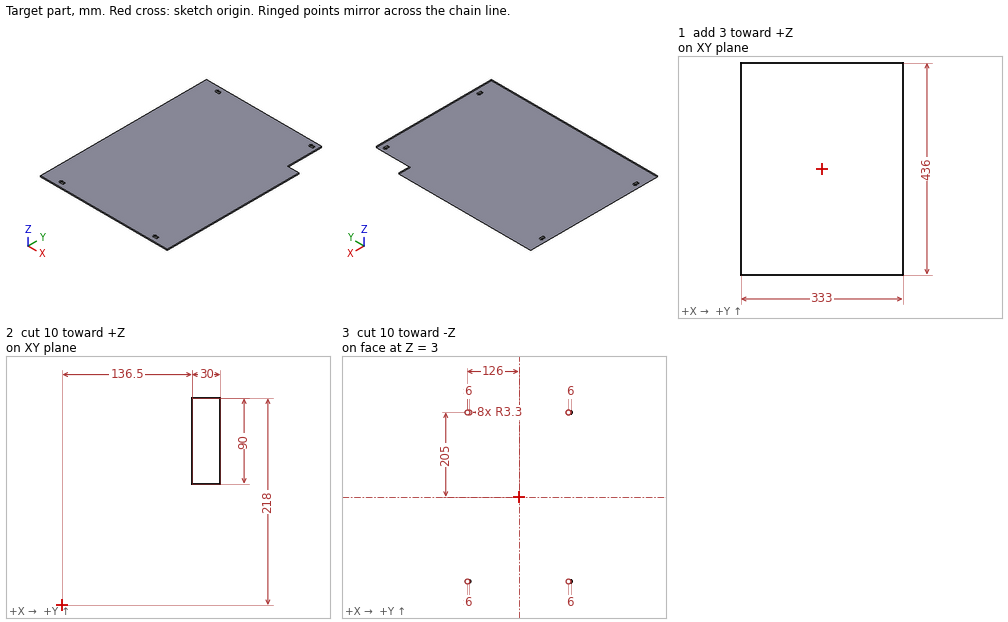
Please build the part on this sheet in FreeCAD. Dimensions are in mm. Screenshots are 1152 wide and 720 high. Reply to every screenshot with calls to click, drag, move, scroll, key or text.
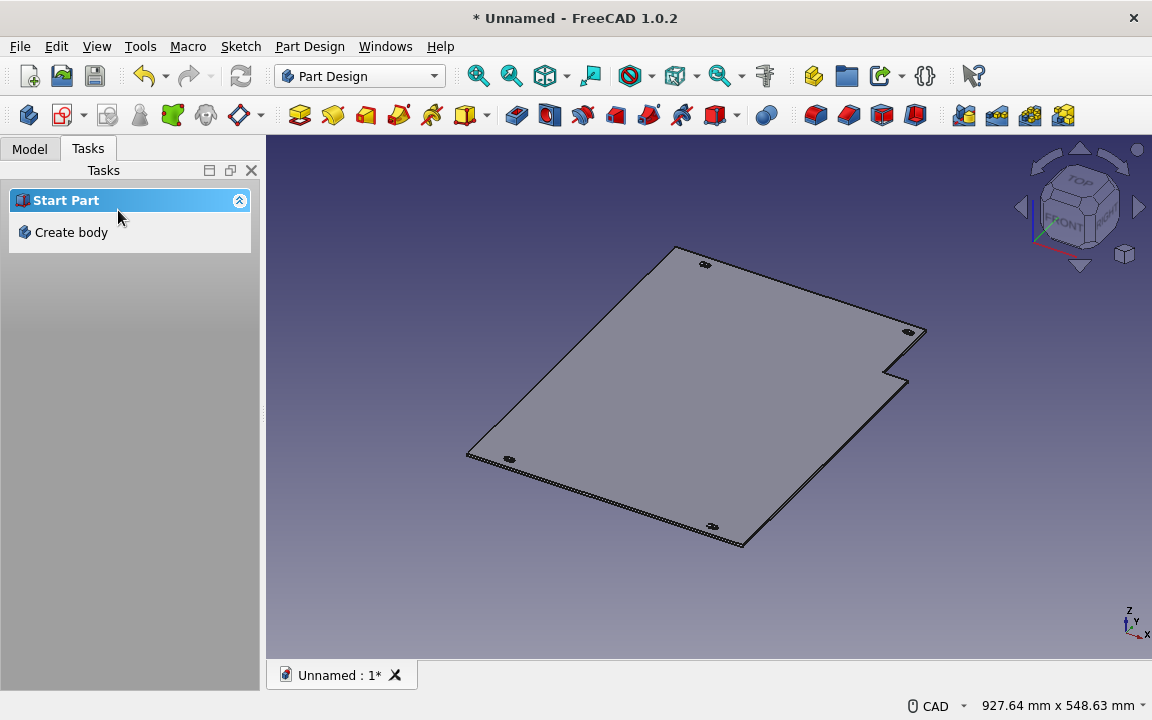
key(0)